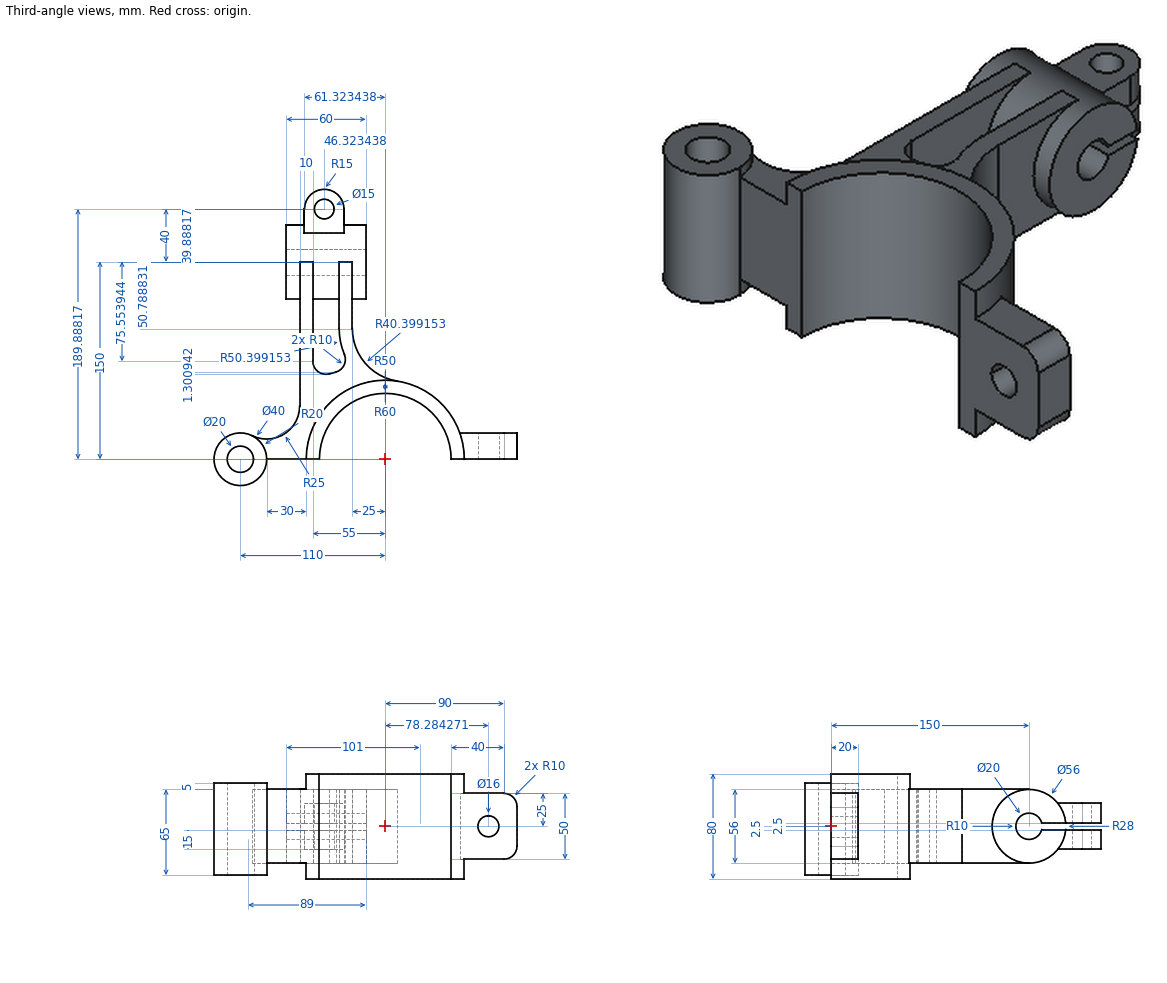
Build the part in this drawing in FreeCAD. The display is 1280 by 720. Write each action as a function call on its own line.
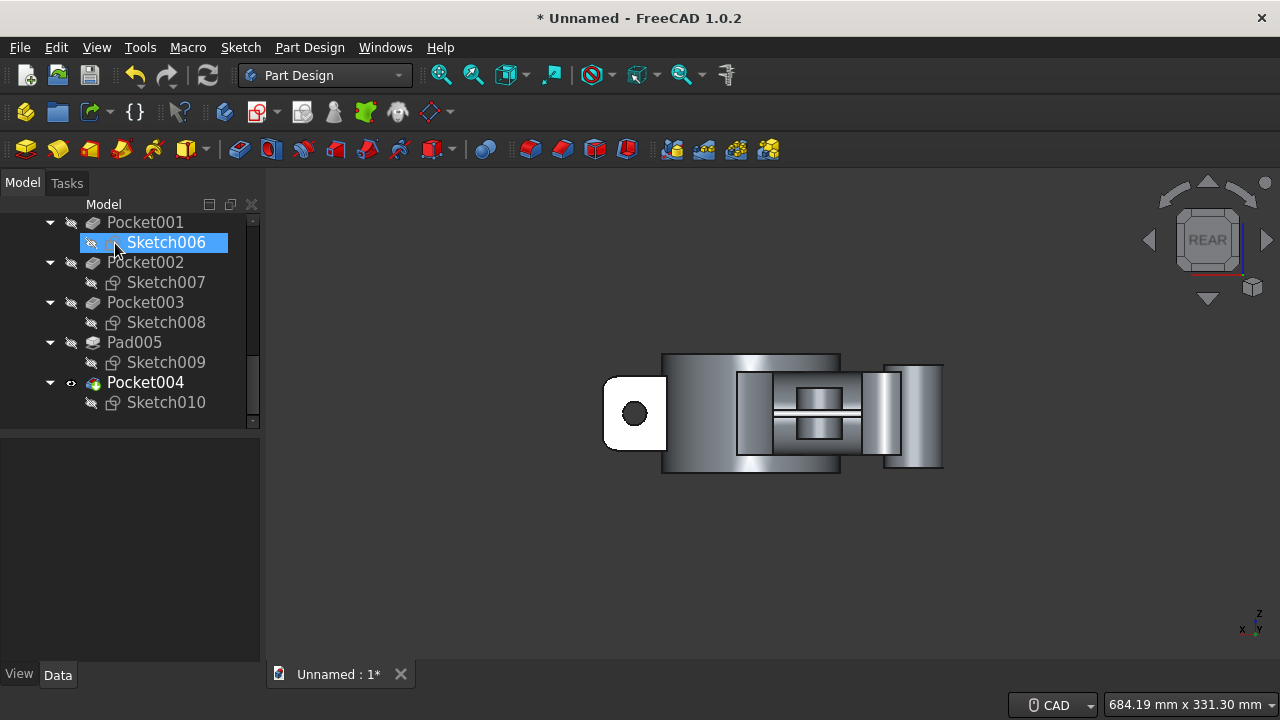
key(0)